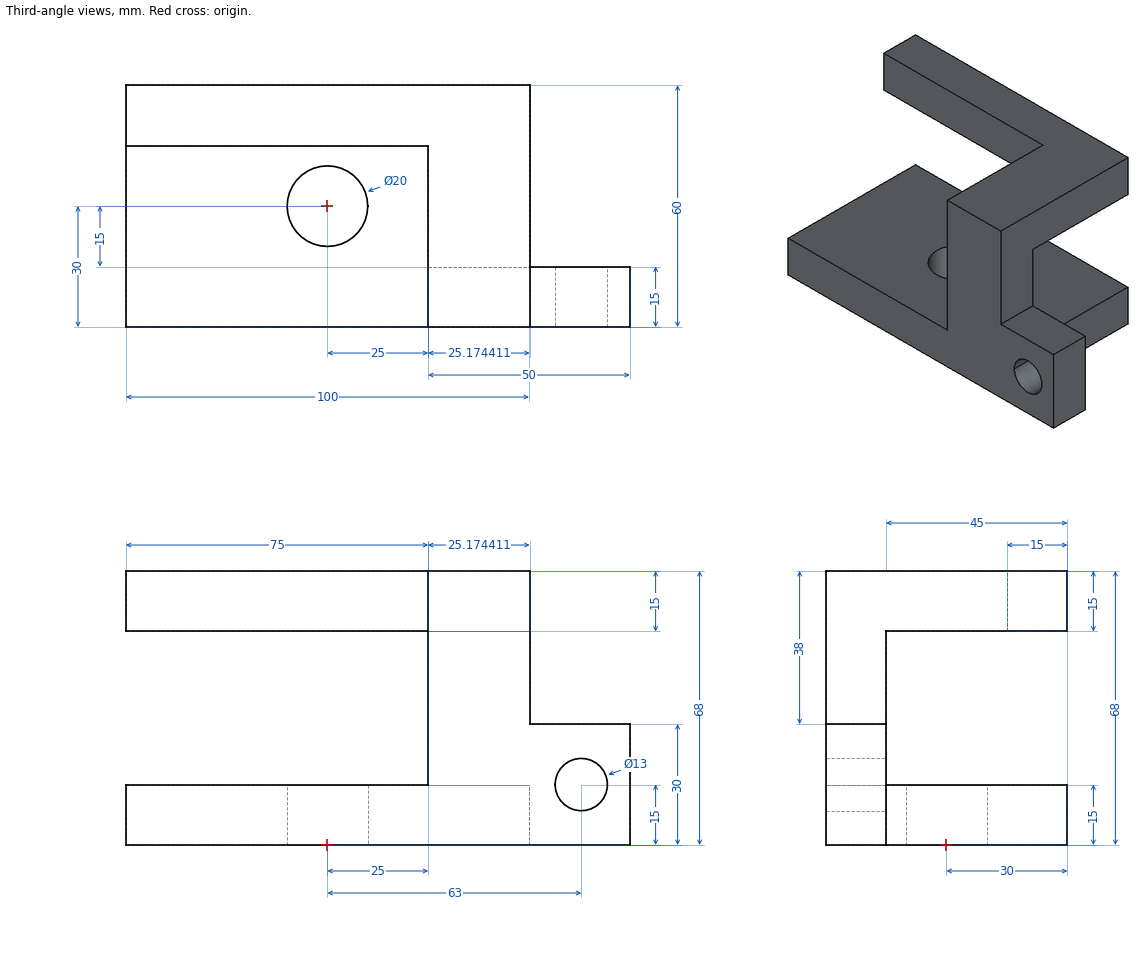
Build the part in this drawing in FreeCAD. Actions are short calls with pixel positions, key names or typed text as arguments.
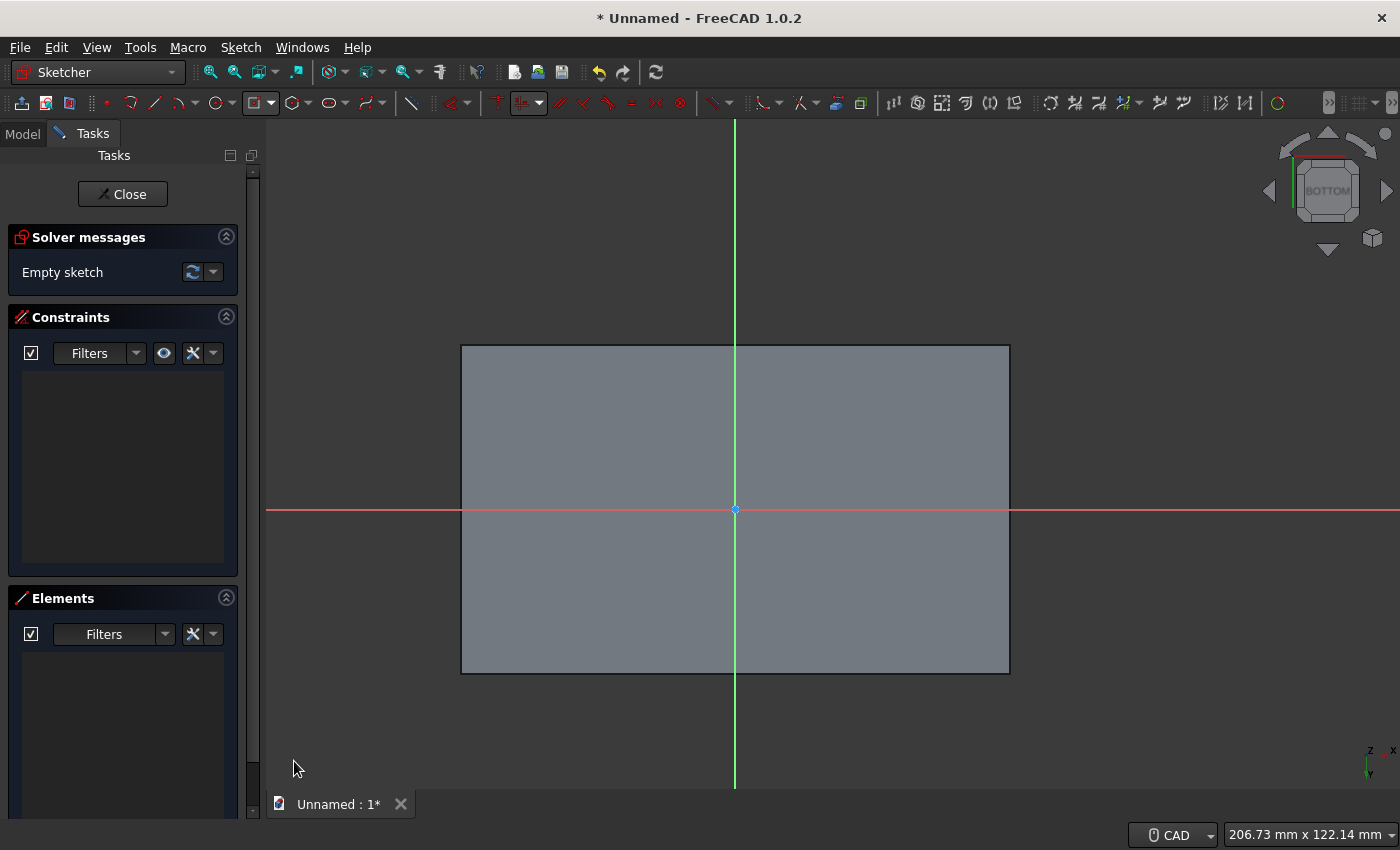
scroll(1235, 374, up, 2)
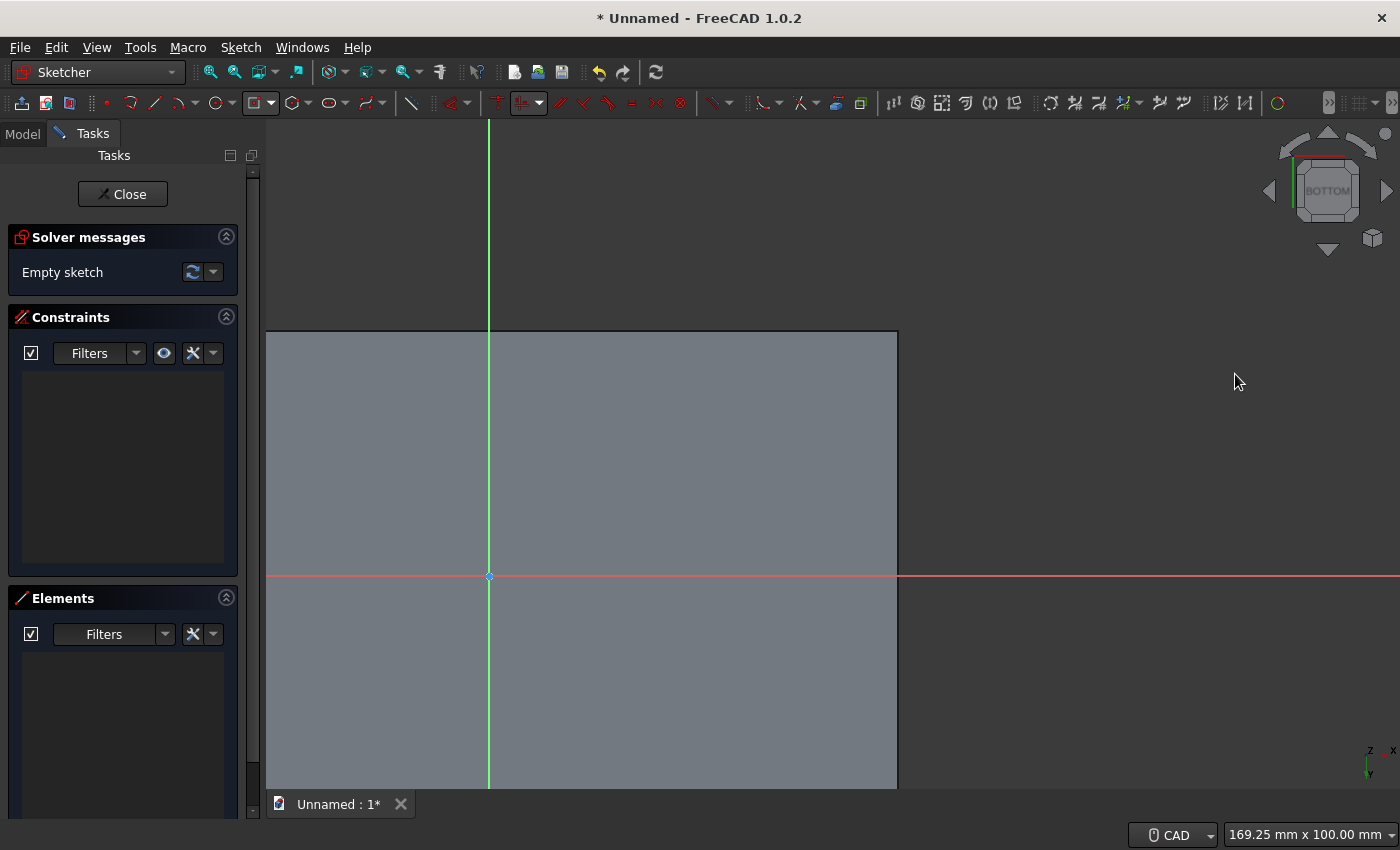
key(g)
key(r)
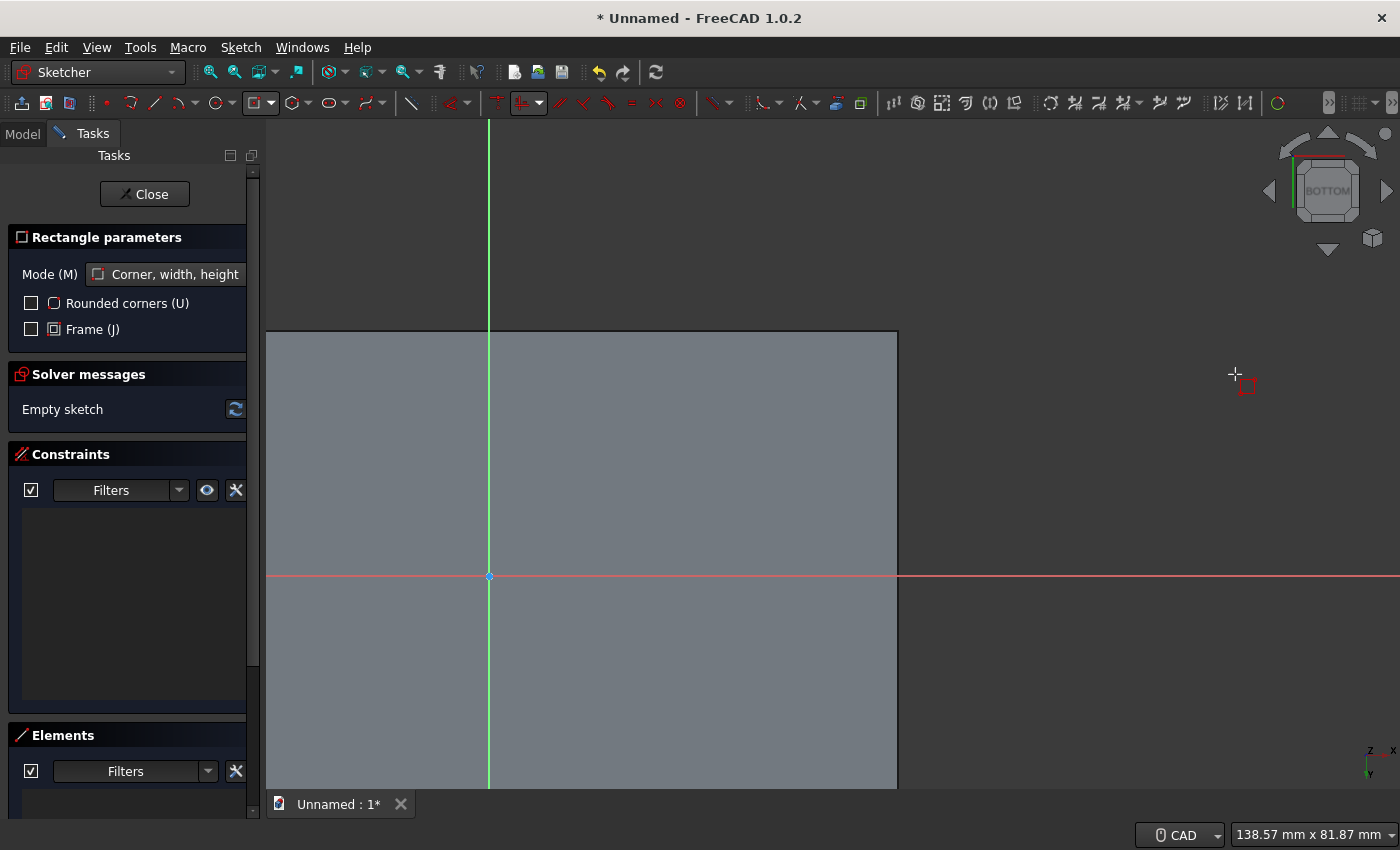
click(694, 331)
move(1103, 454)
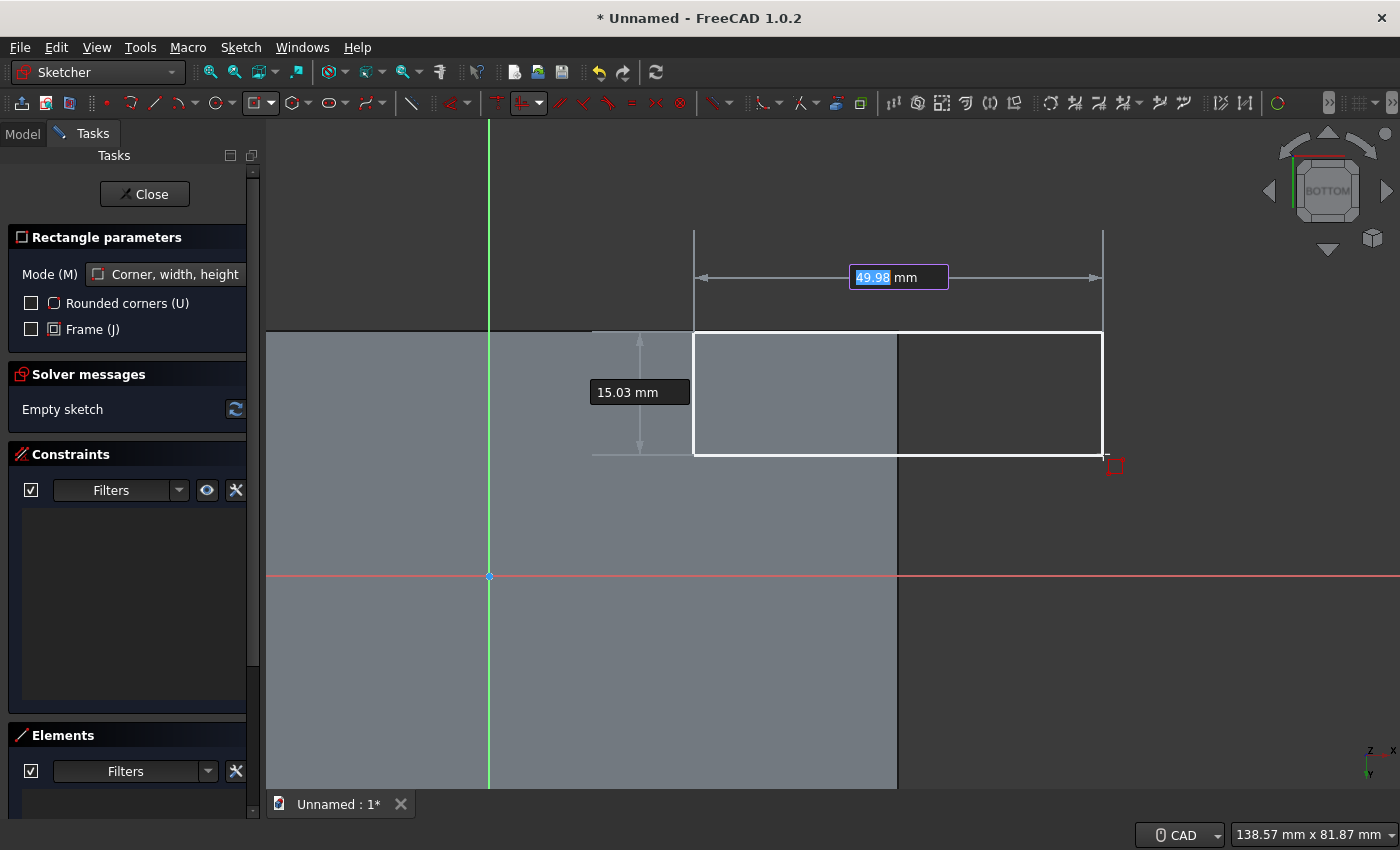
text(50)
key(Tab)
text(15)
key(Return)
key(Escape)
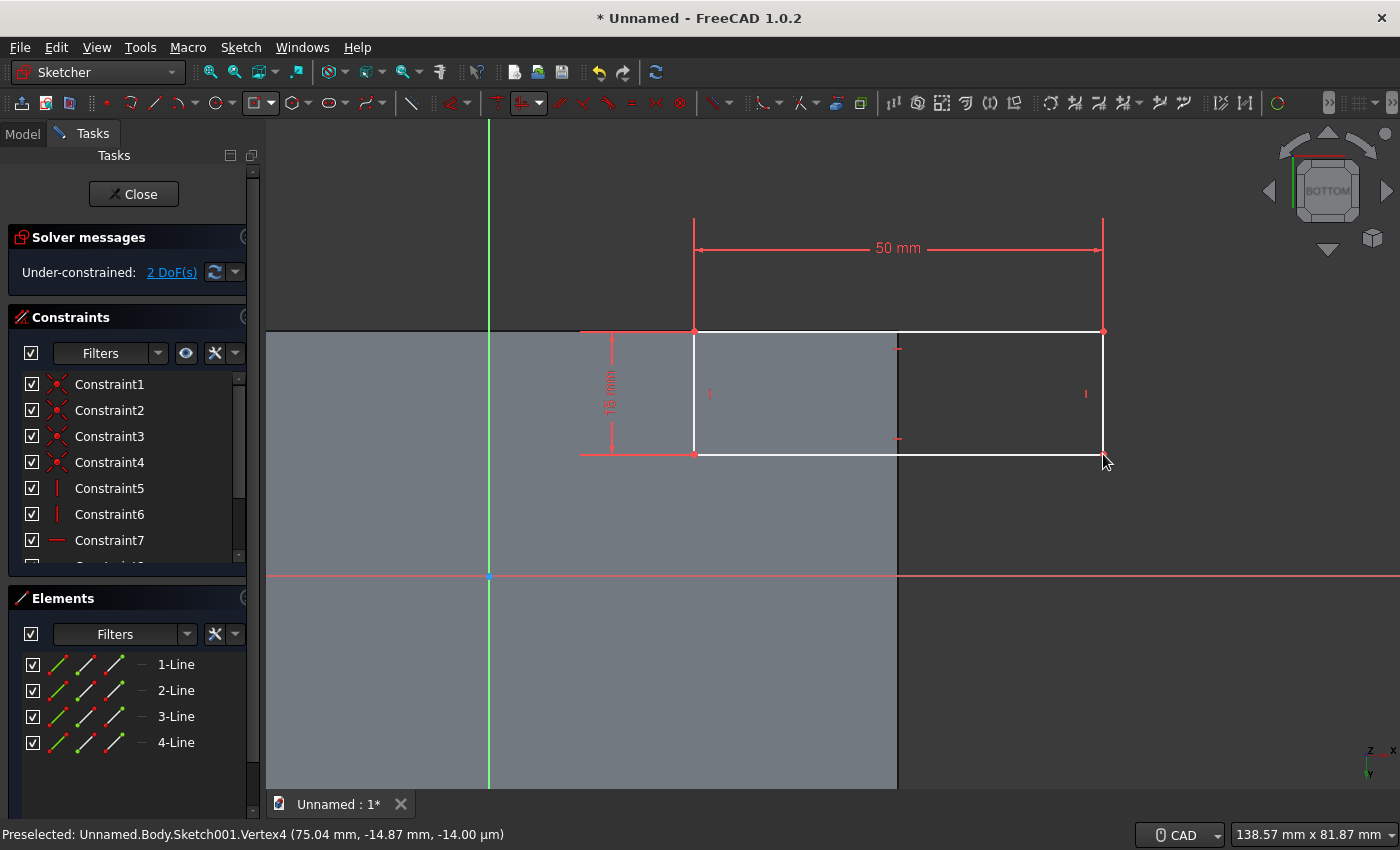
click(450, 104)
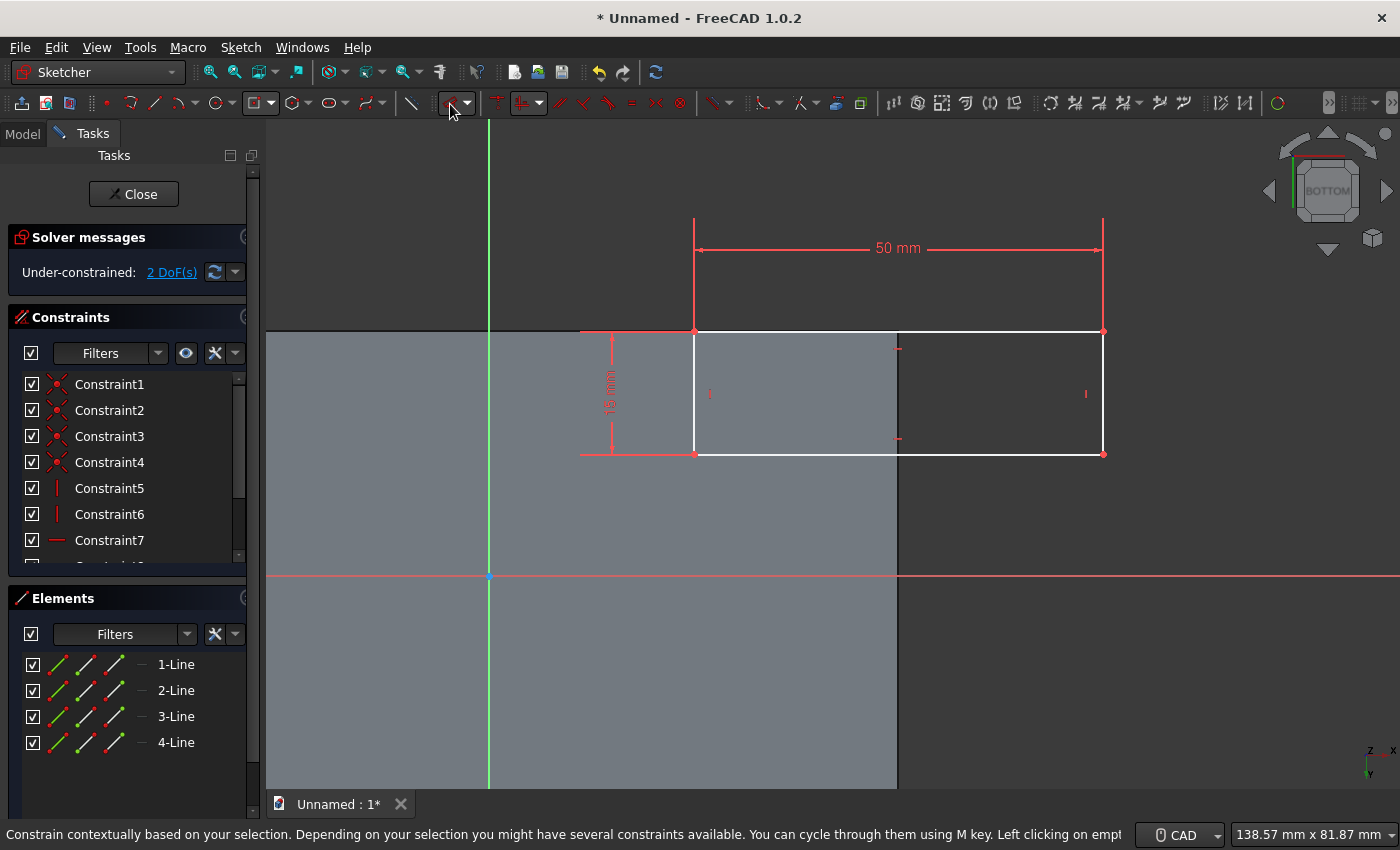
click(694, 332)
click(592, 610)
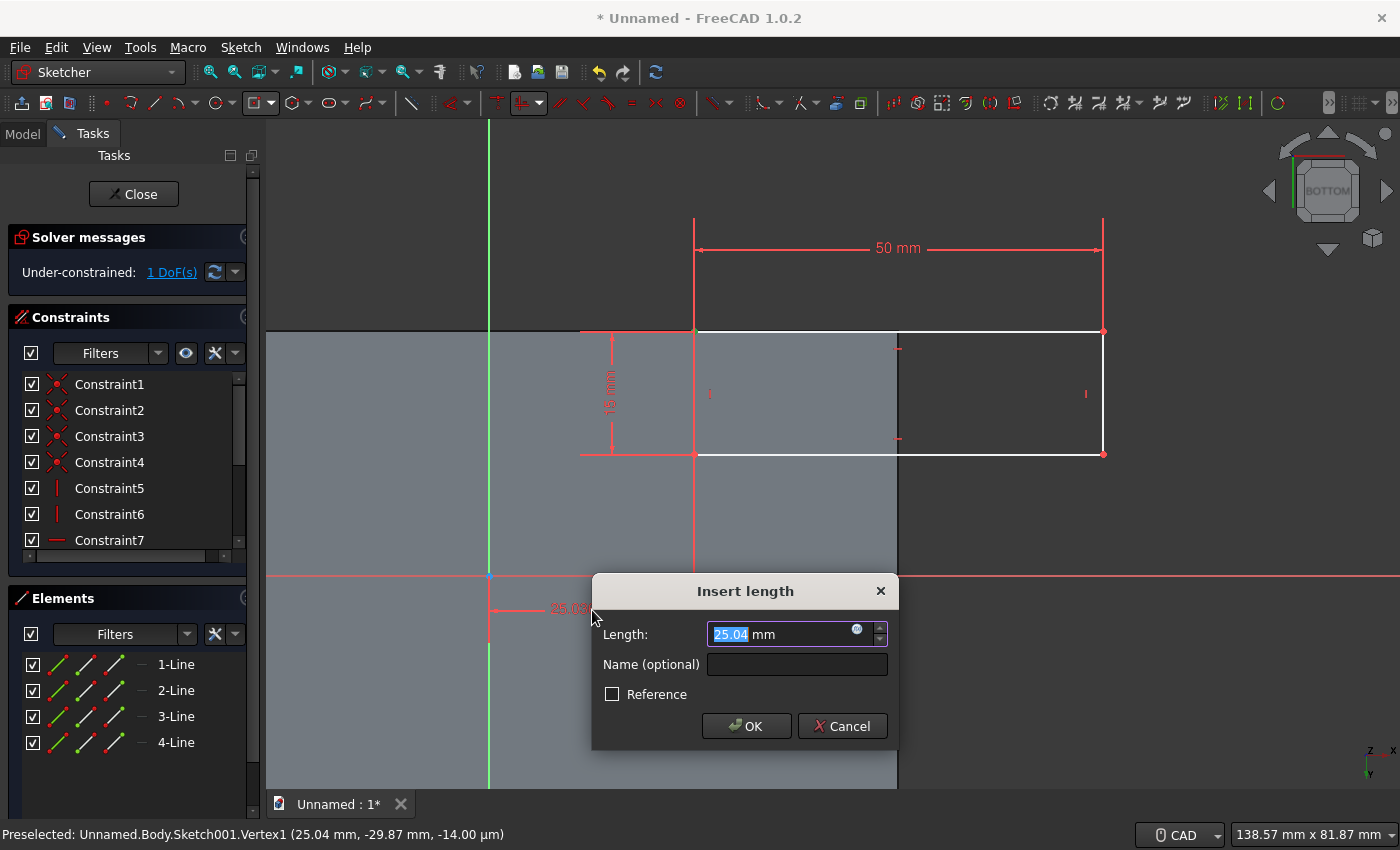
text(25)
key(Return)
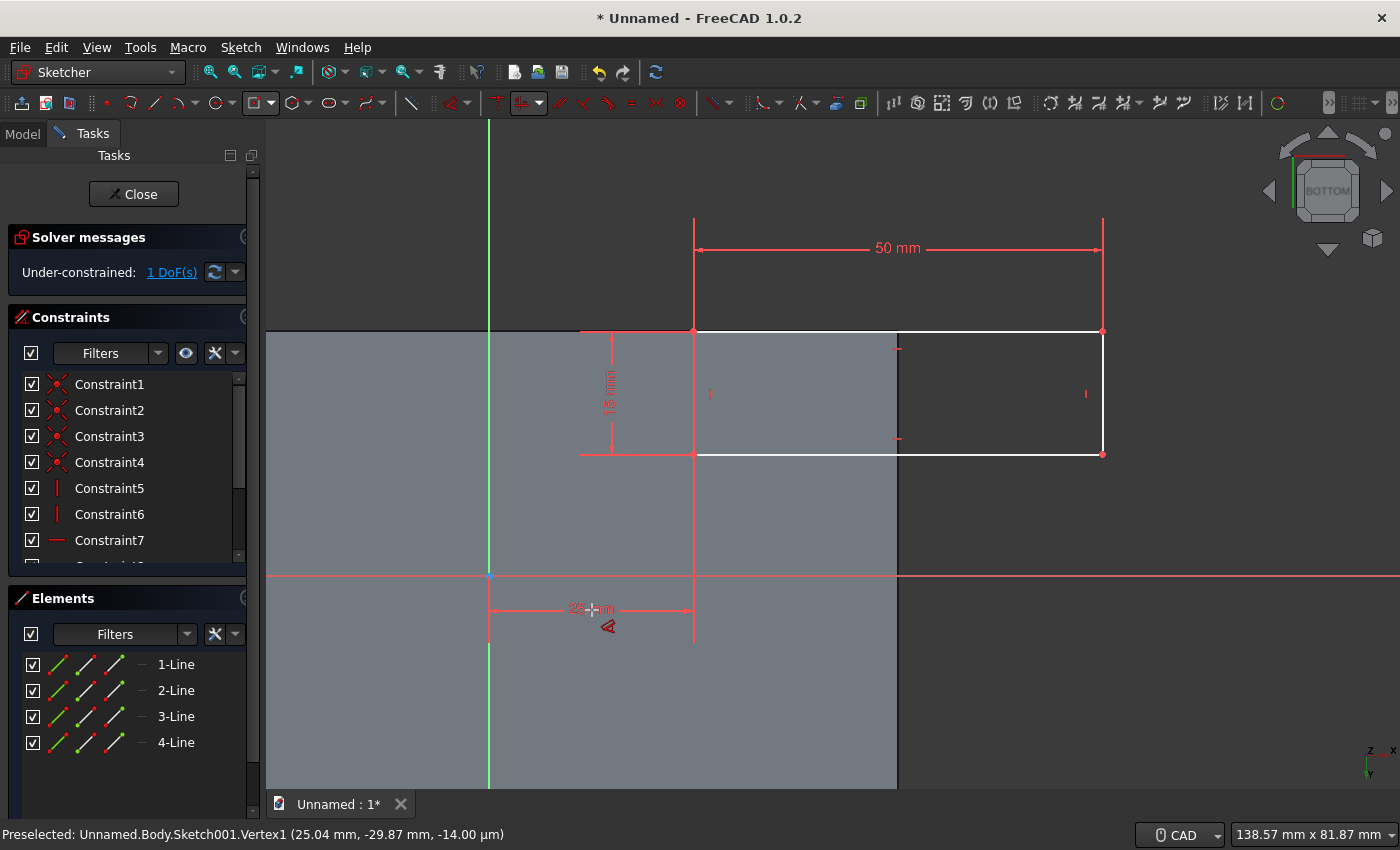
click(694, 332)
click(455, 454)